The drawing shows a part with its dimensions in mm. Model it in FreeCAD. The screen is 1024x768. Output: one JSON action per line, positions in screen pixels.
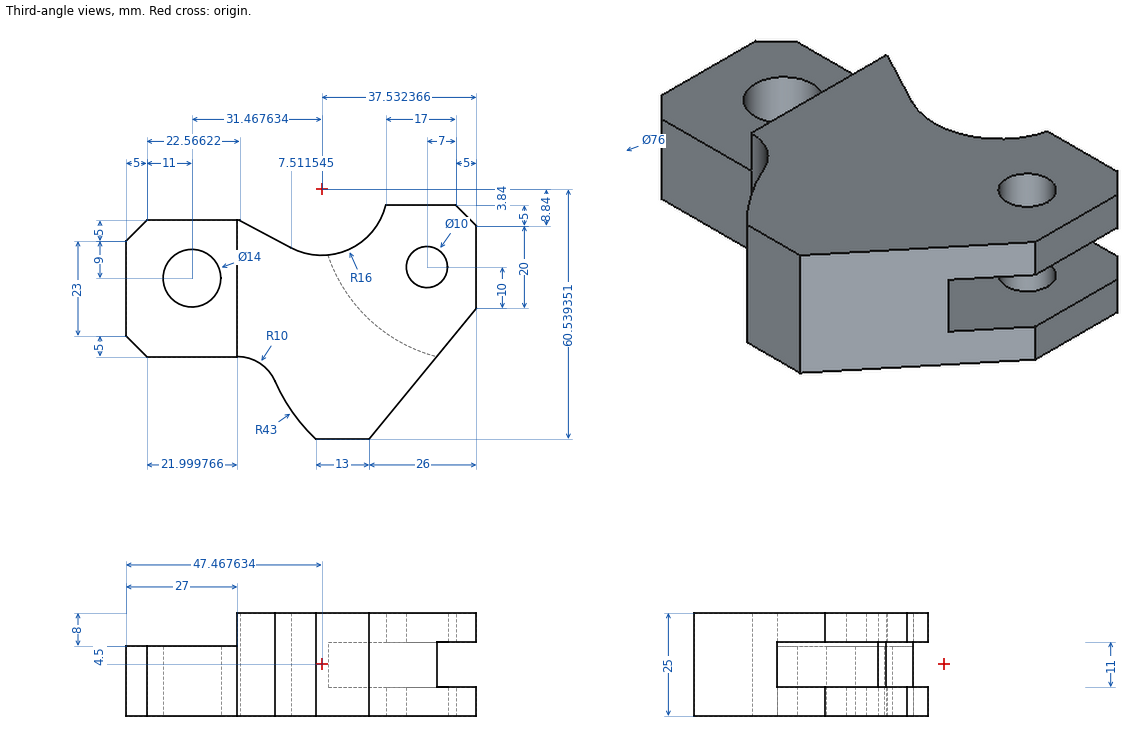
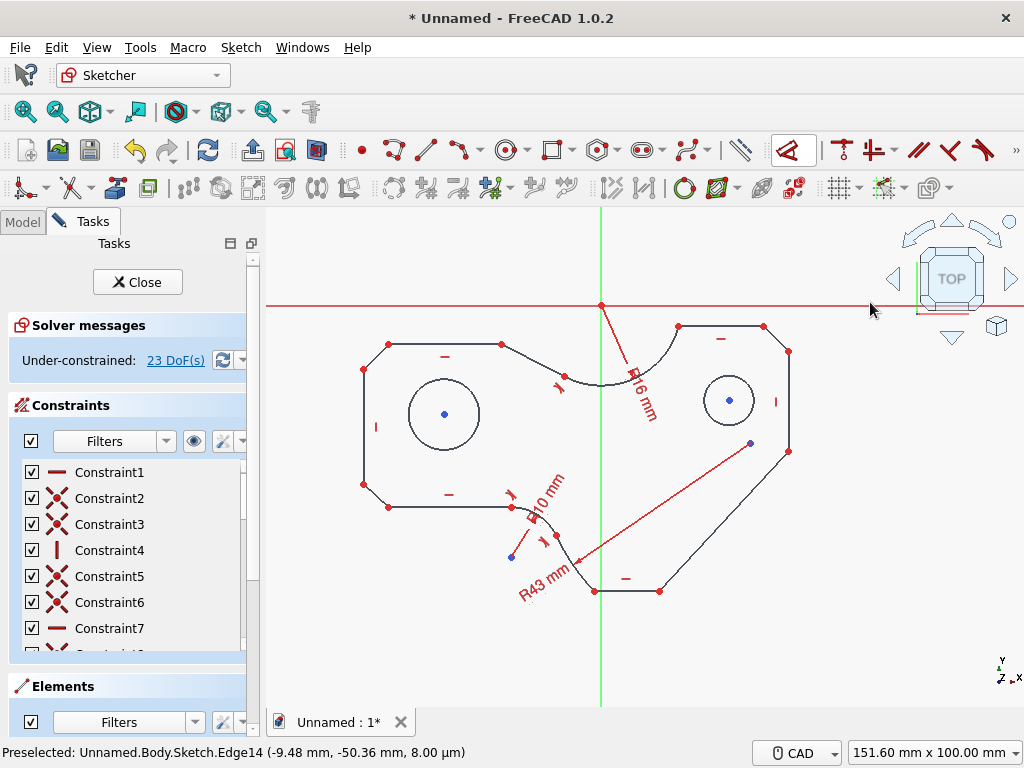
{"action": "left_click", "coordinate": [469, 389]}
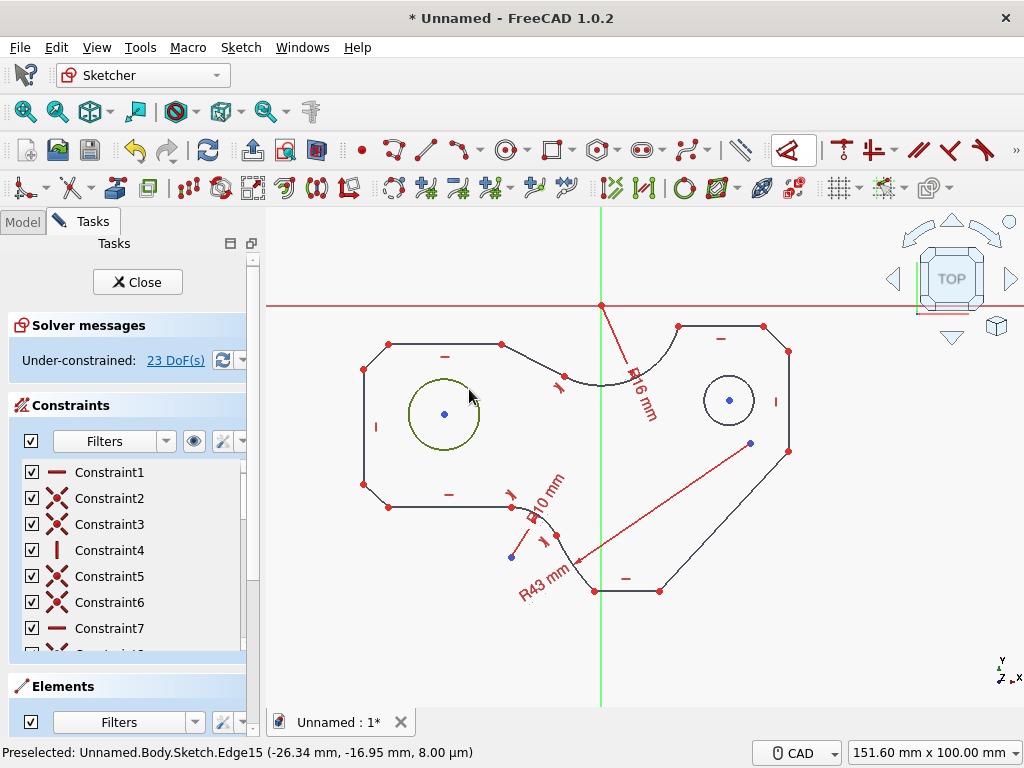
{"action": "key", "text": "k o"}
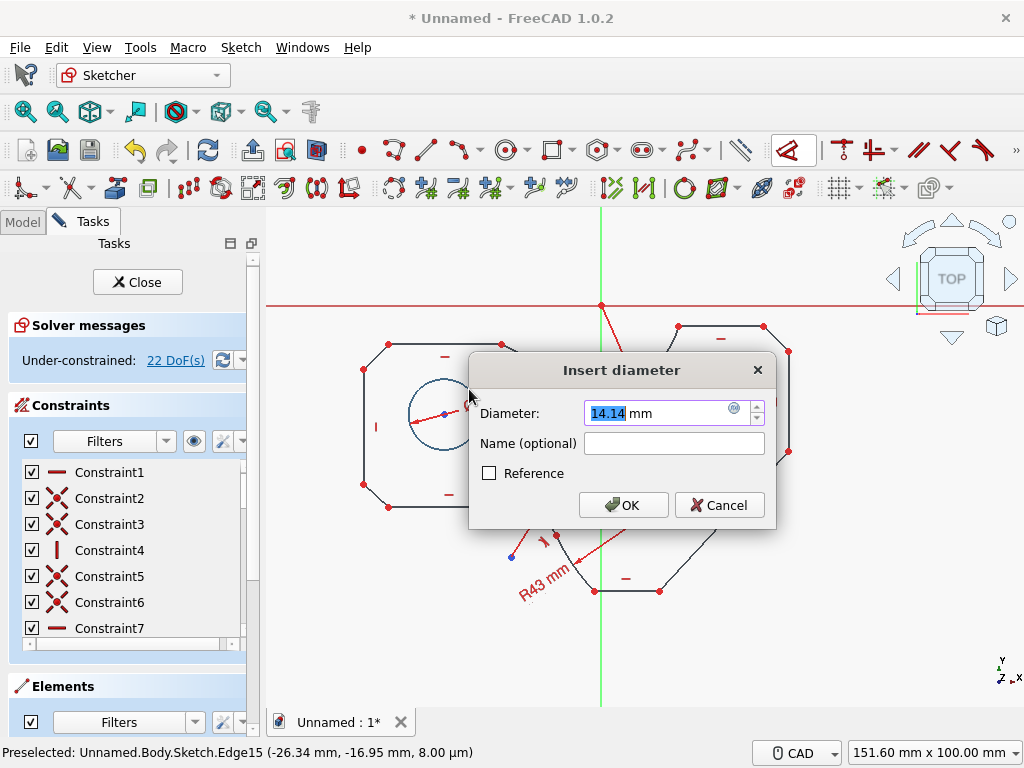
{"action": "type", "text": "14"}
{"action": "key", "text": "Return"}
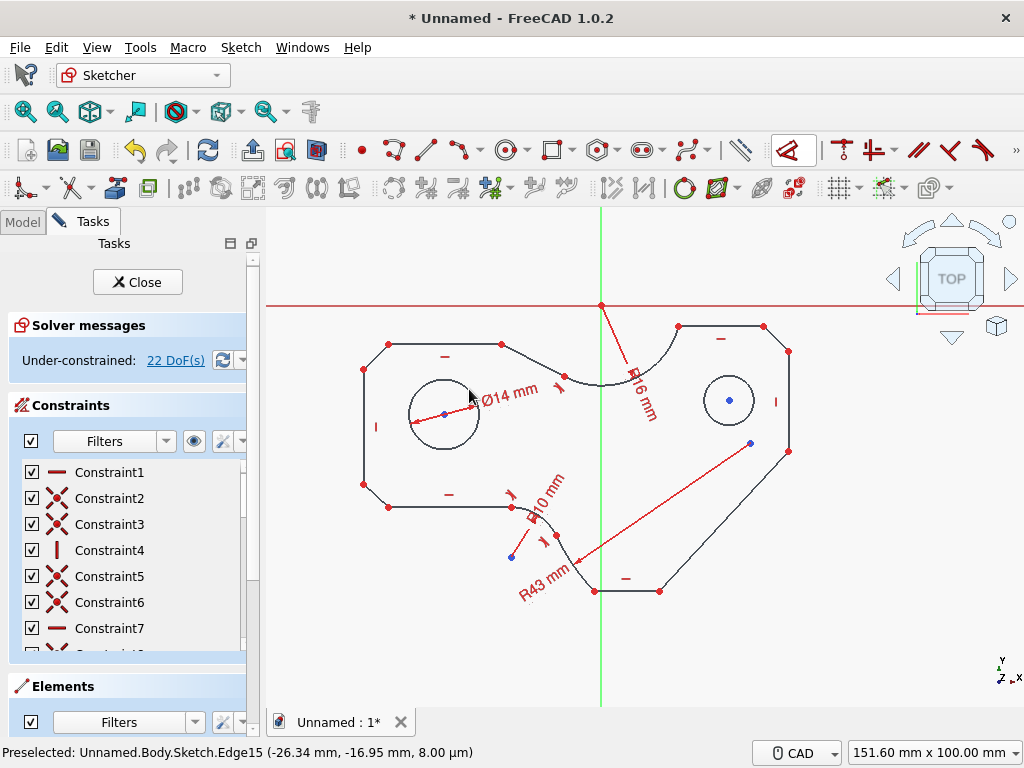
{"action": "left_click", "coordinate": [746, 383]}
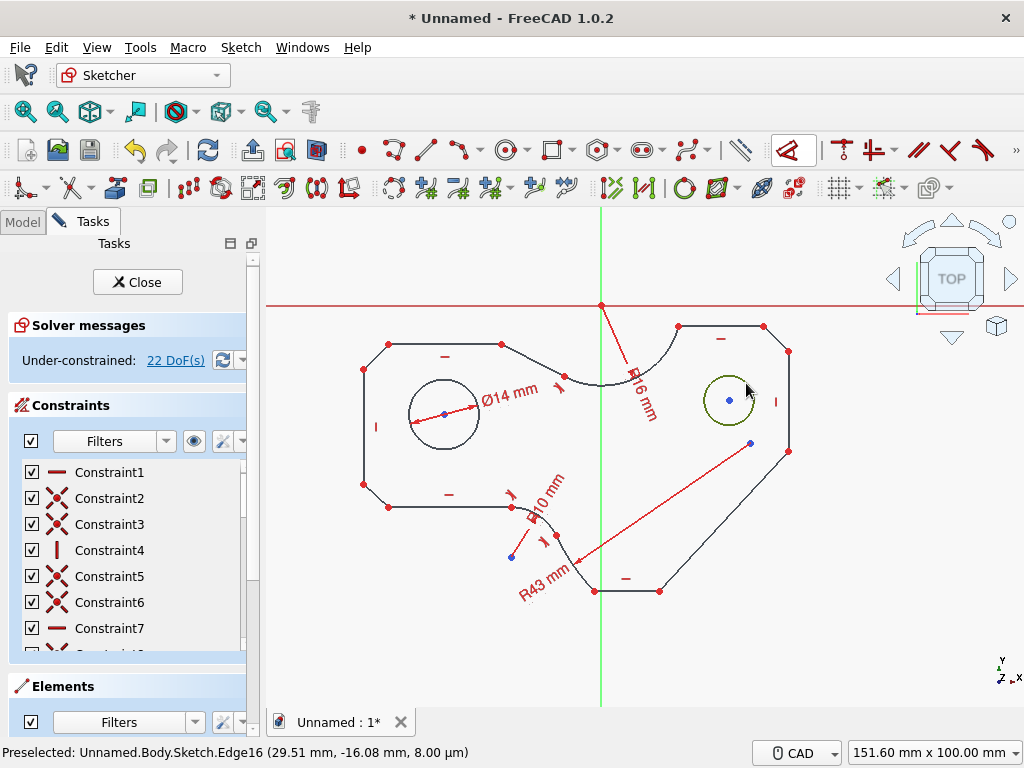
{"action": "left_click", "coordinate": [810, 150]}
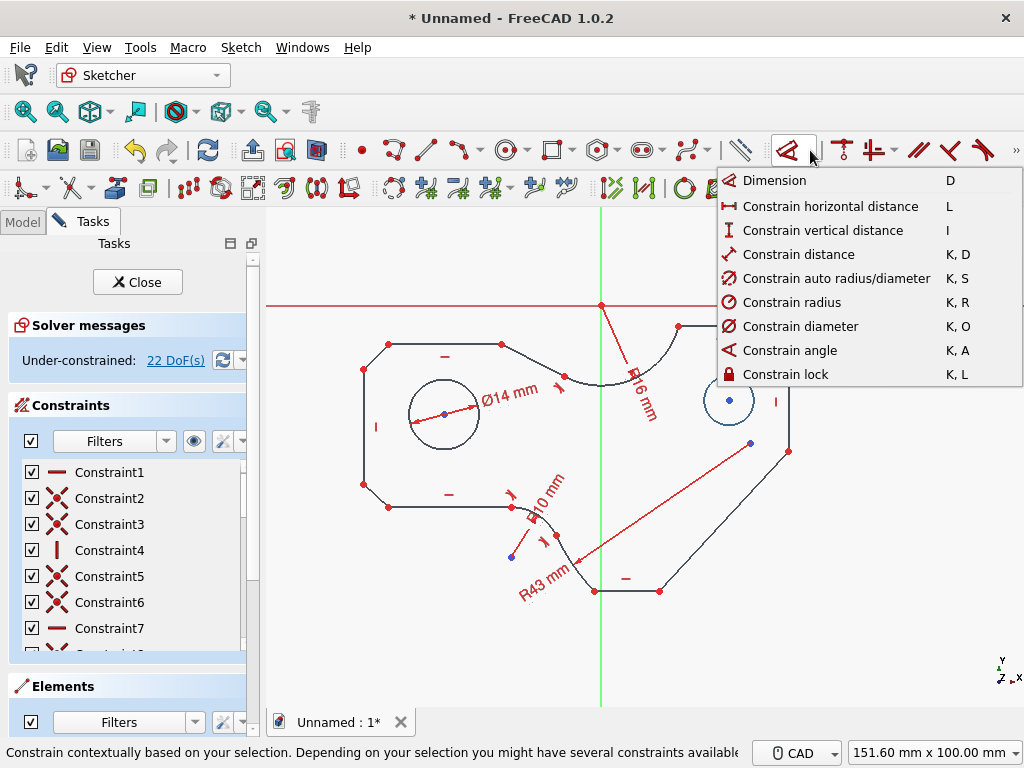
{"action": "left_click", "coordinate": [870, 326]}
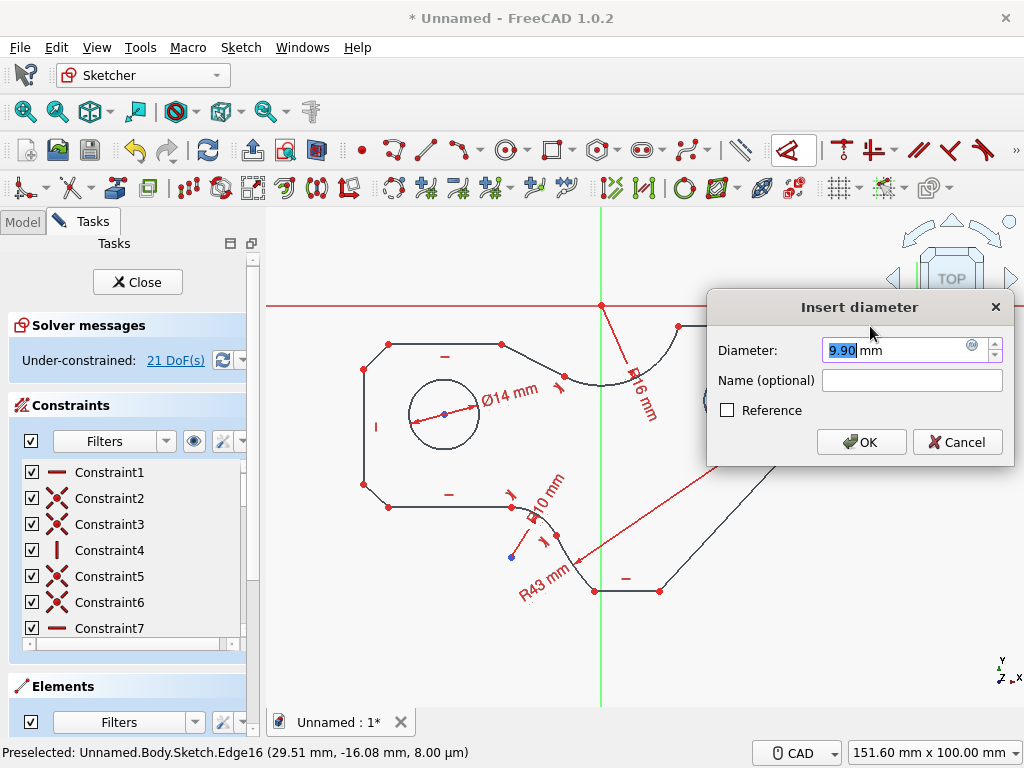
{"action": "type", "text": "10"}
{"action": "key", "text": "Return"}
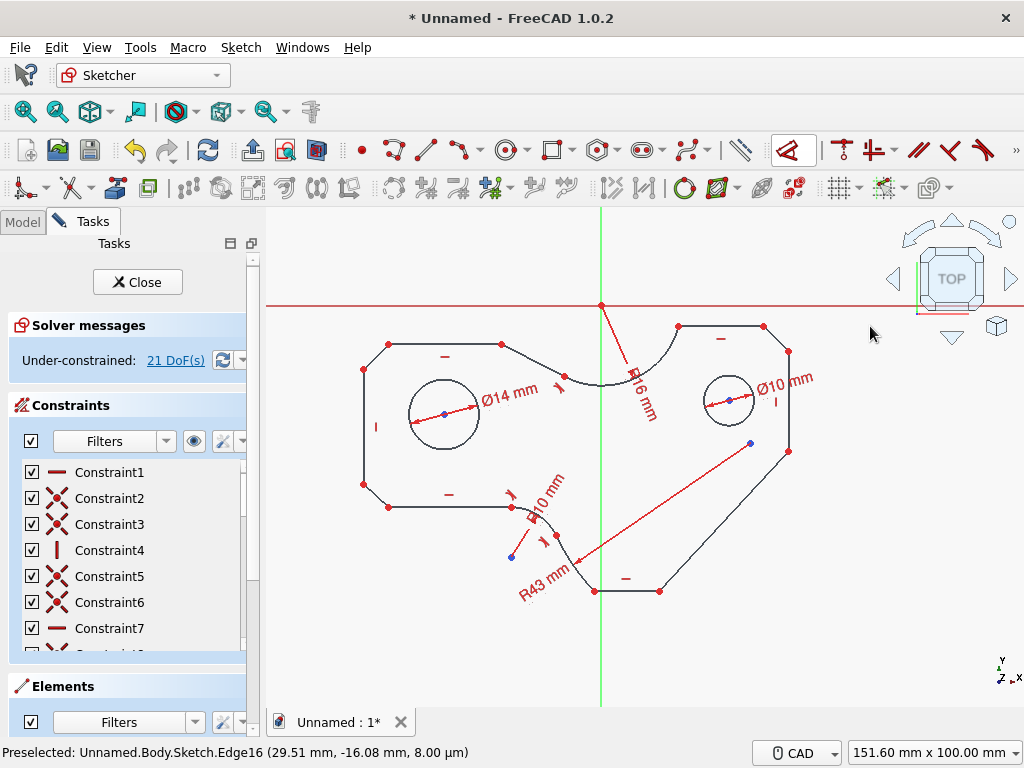
{"action": "left_click", "coordinate": [614, 591]}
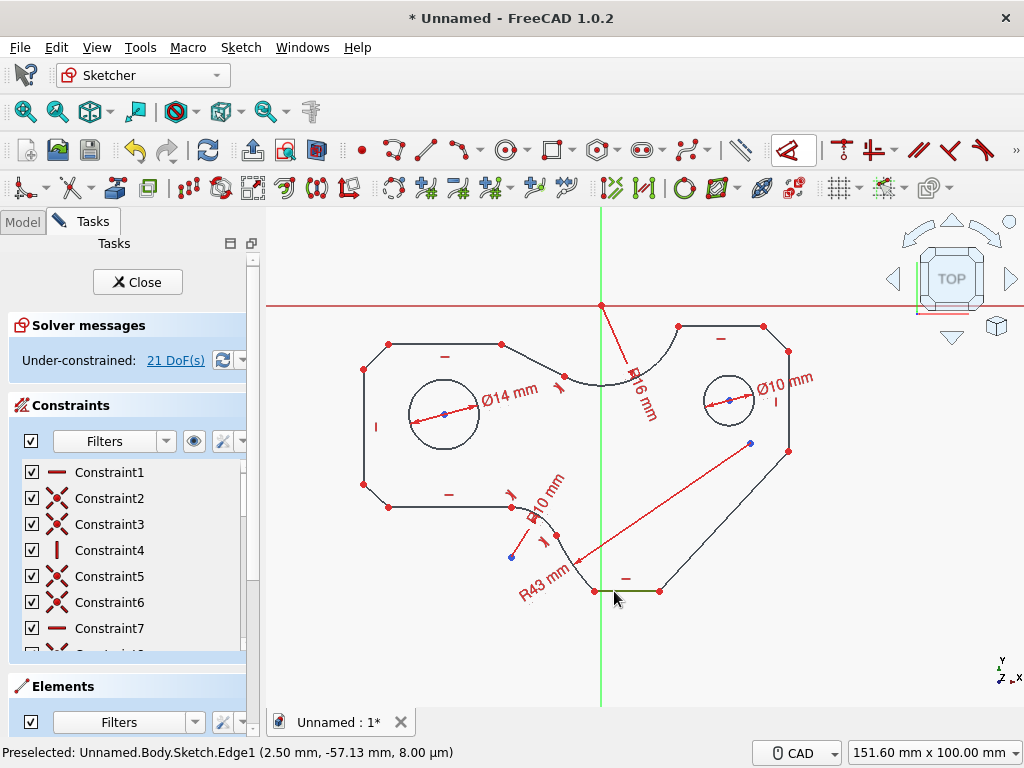
{"action": "left_click", "coordinate": [810, 150]}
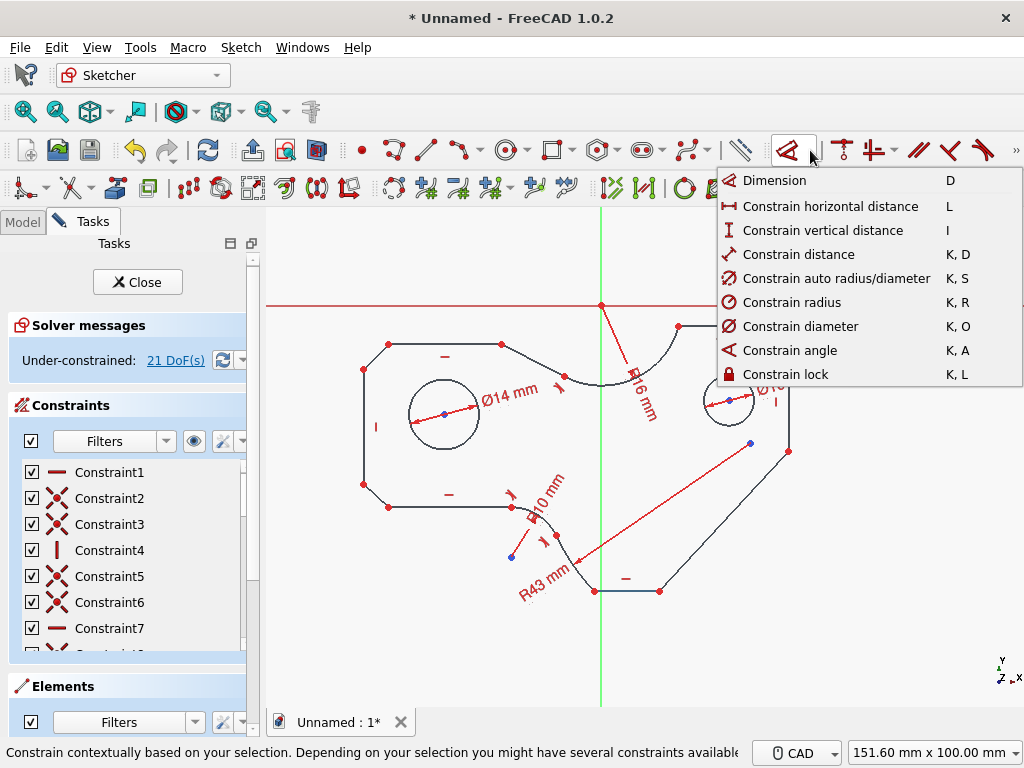
{"action": "left_click", "coordinate": [870, 206]}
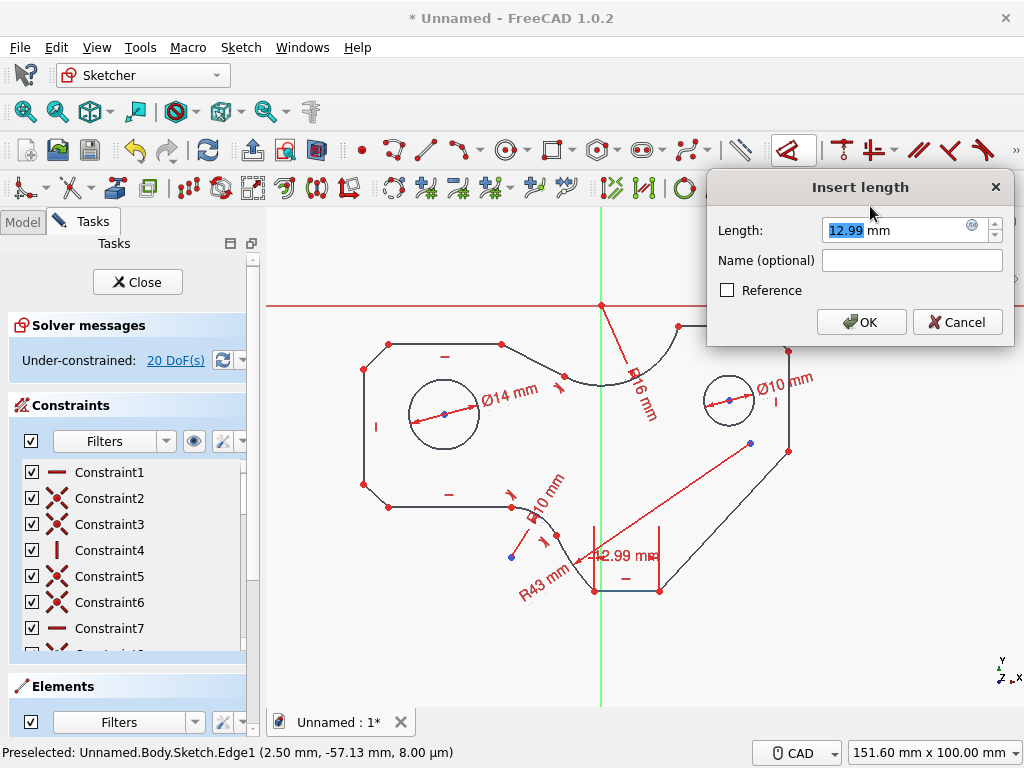
{"action": "type", "text": "13"}
{"action": "key", "text": "Return"}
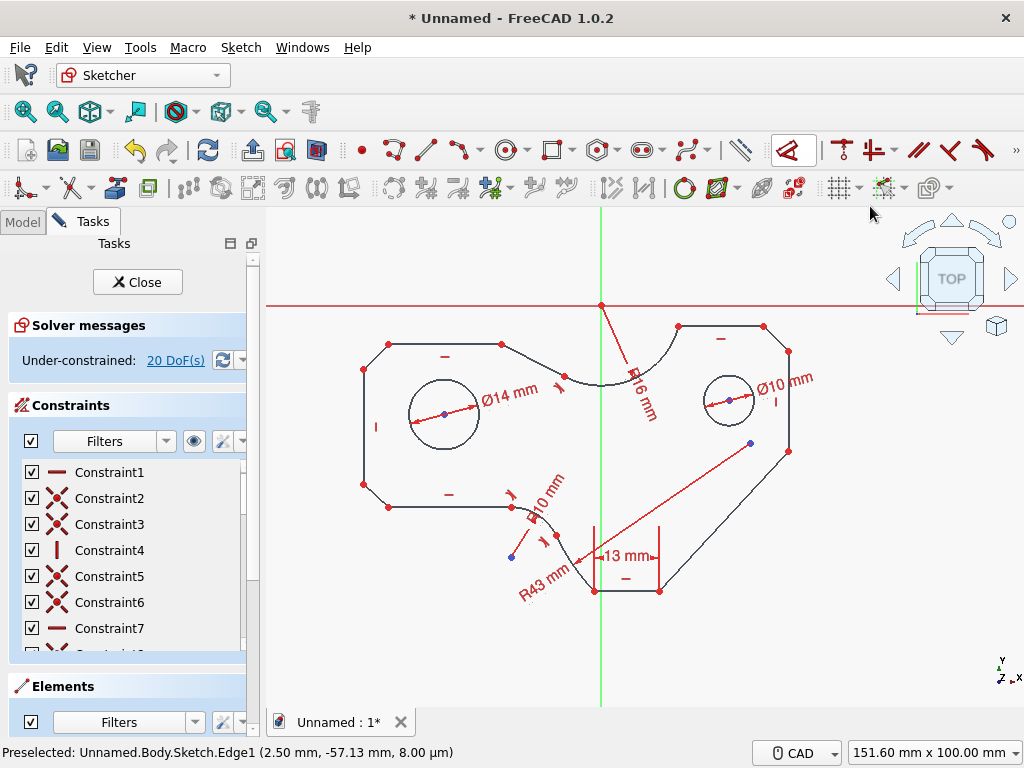
{"action": "left_click", "coordinate": [789, 421]}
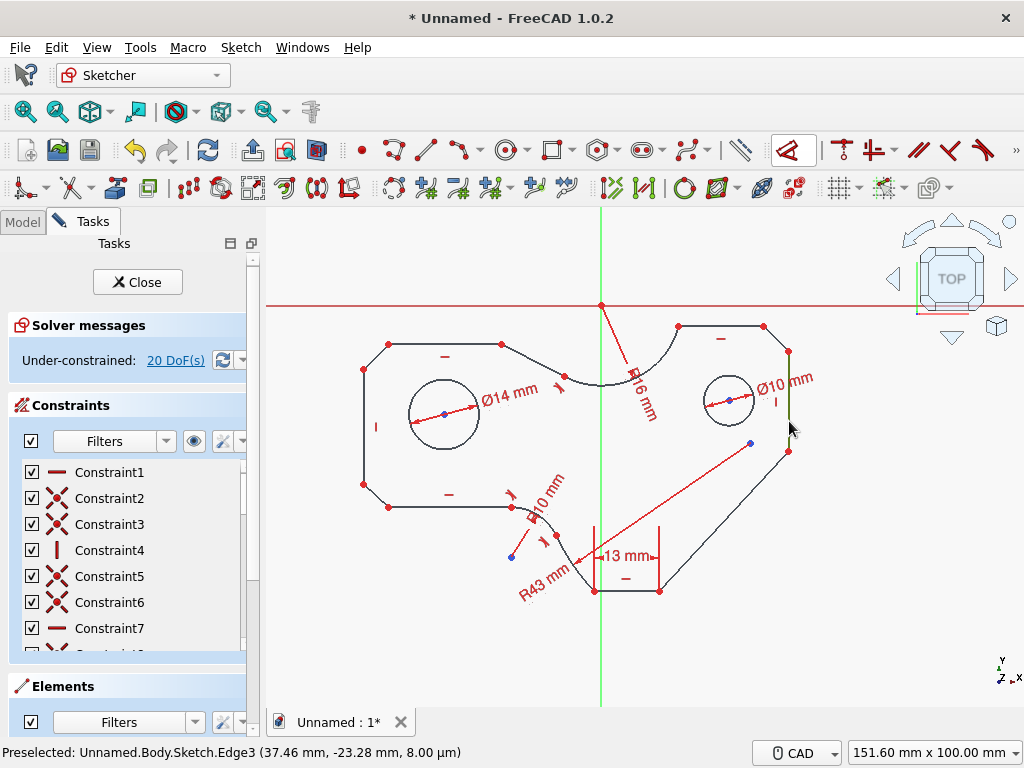
{"action": "left_click", "coordinate": [810, 150]}